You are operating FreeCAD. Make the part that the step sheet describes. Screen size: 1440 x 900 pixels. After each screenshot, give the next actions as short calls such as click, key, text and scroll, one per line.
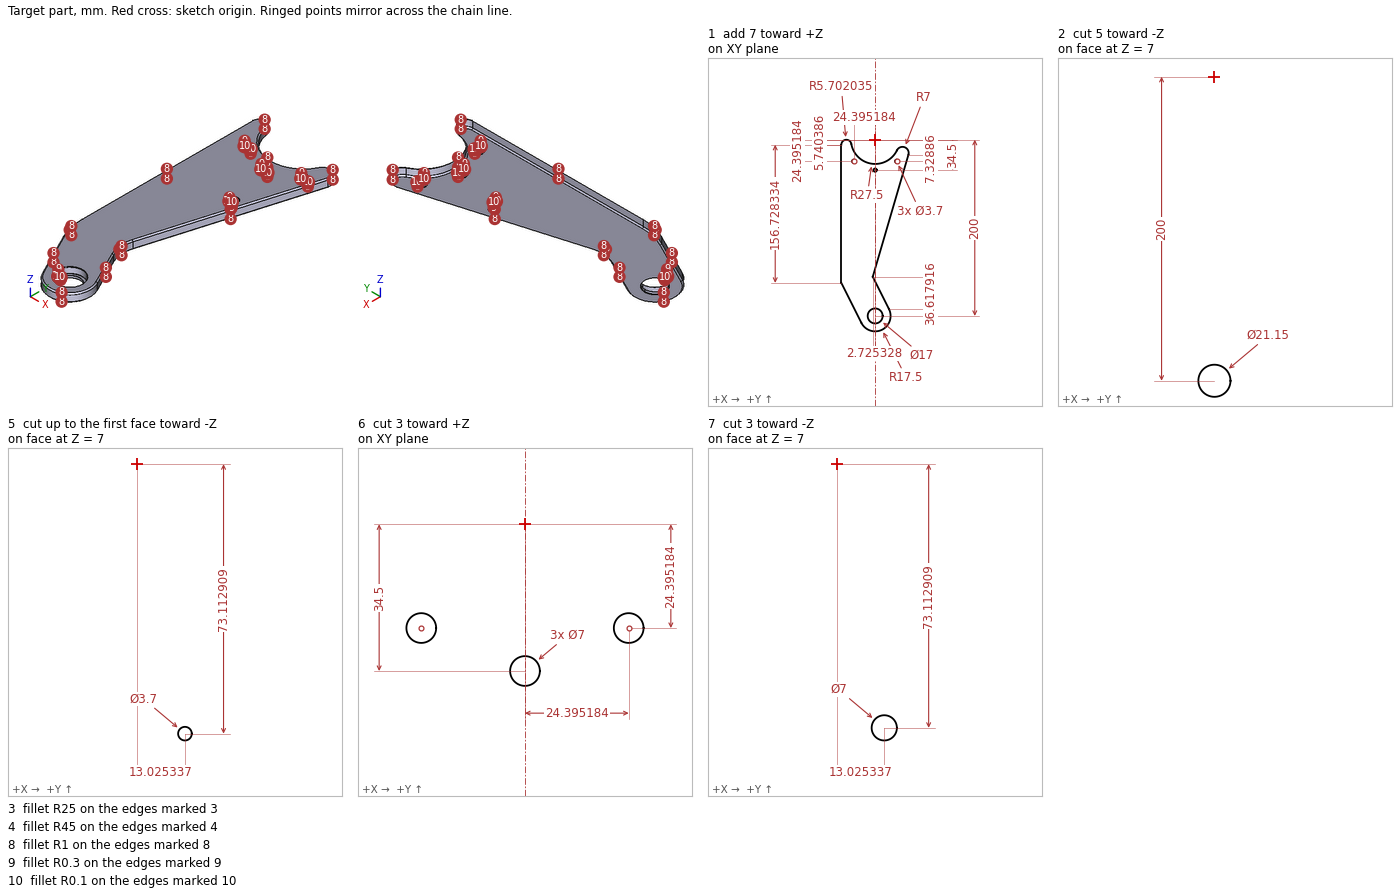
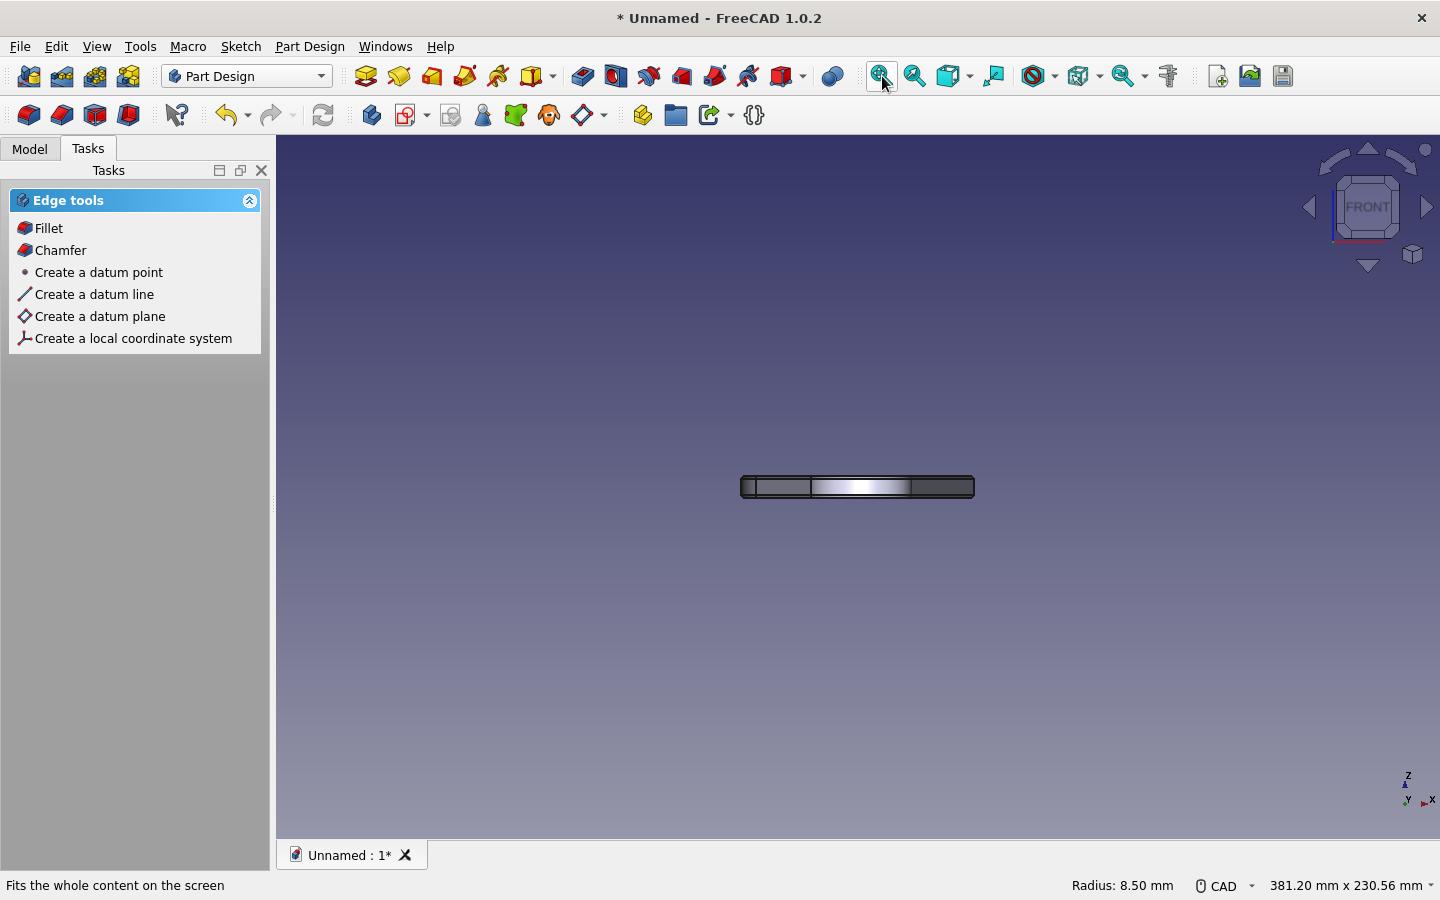
key(3)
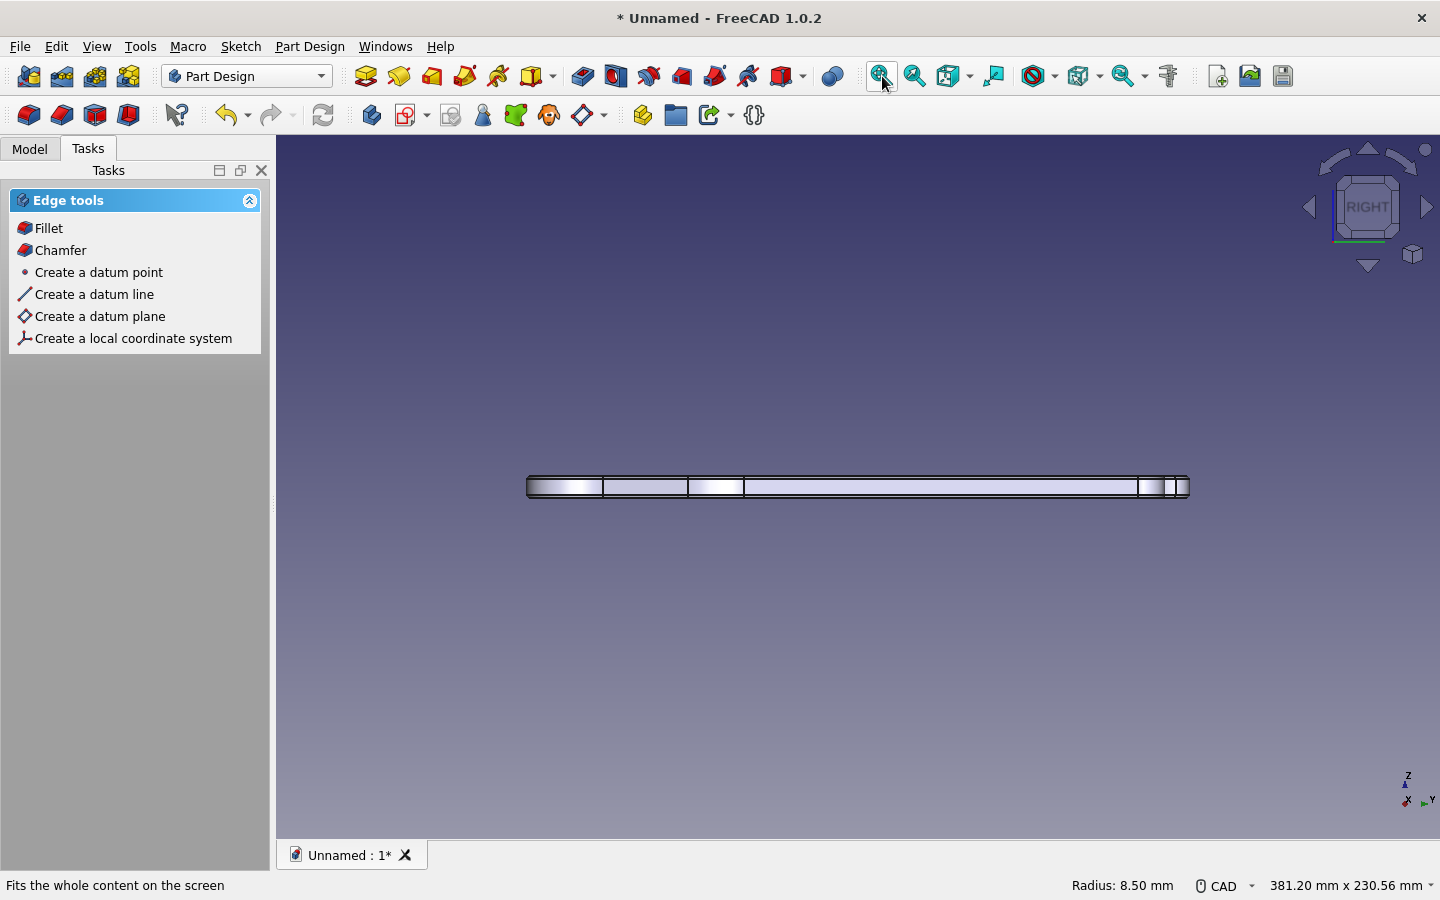
key(5)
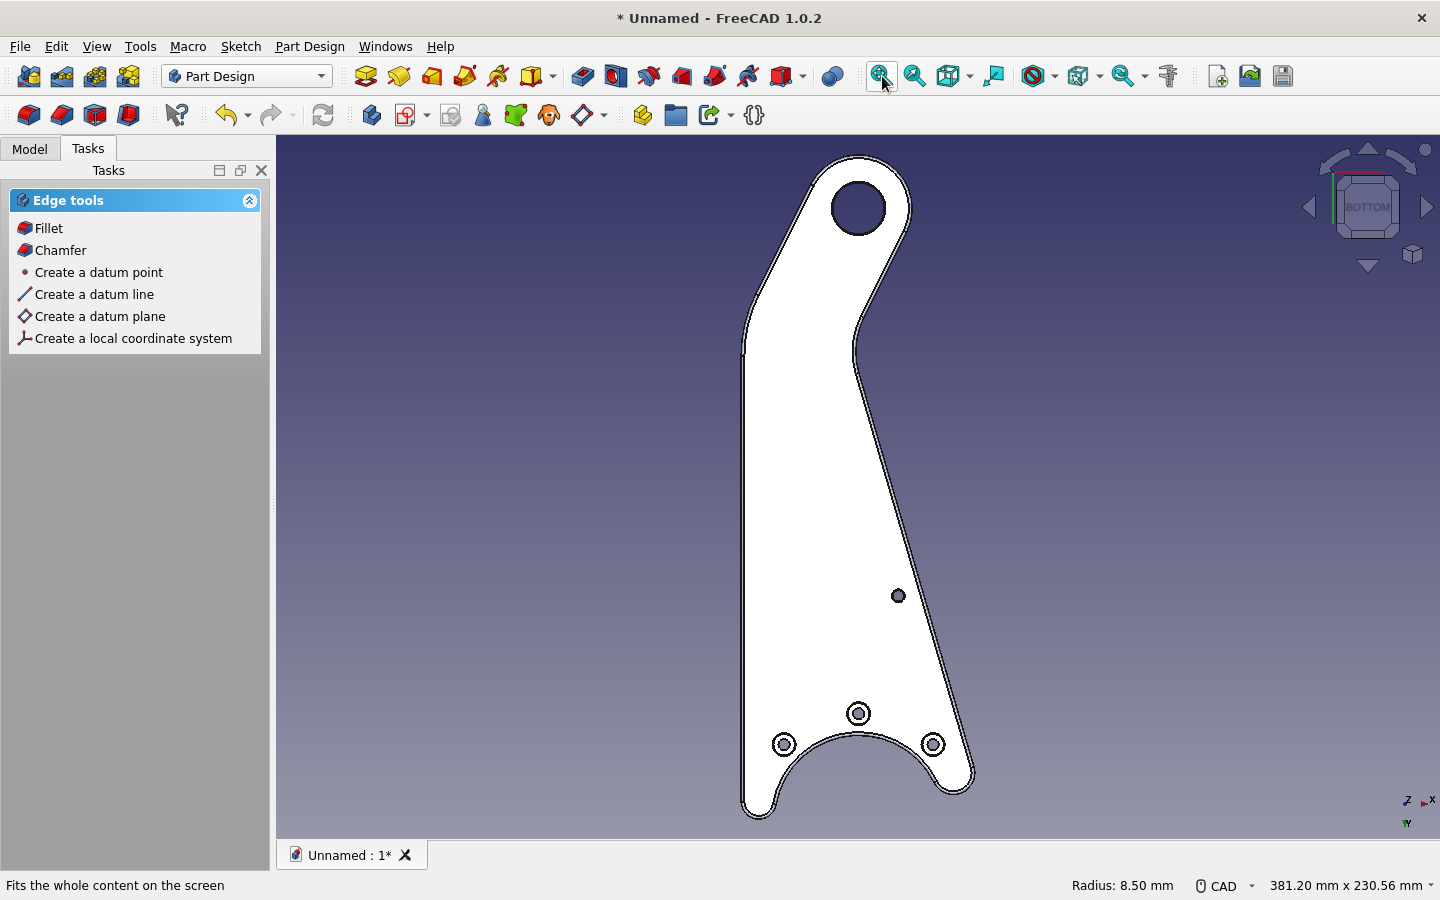
key(4)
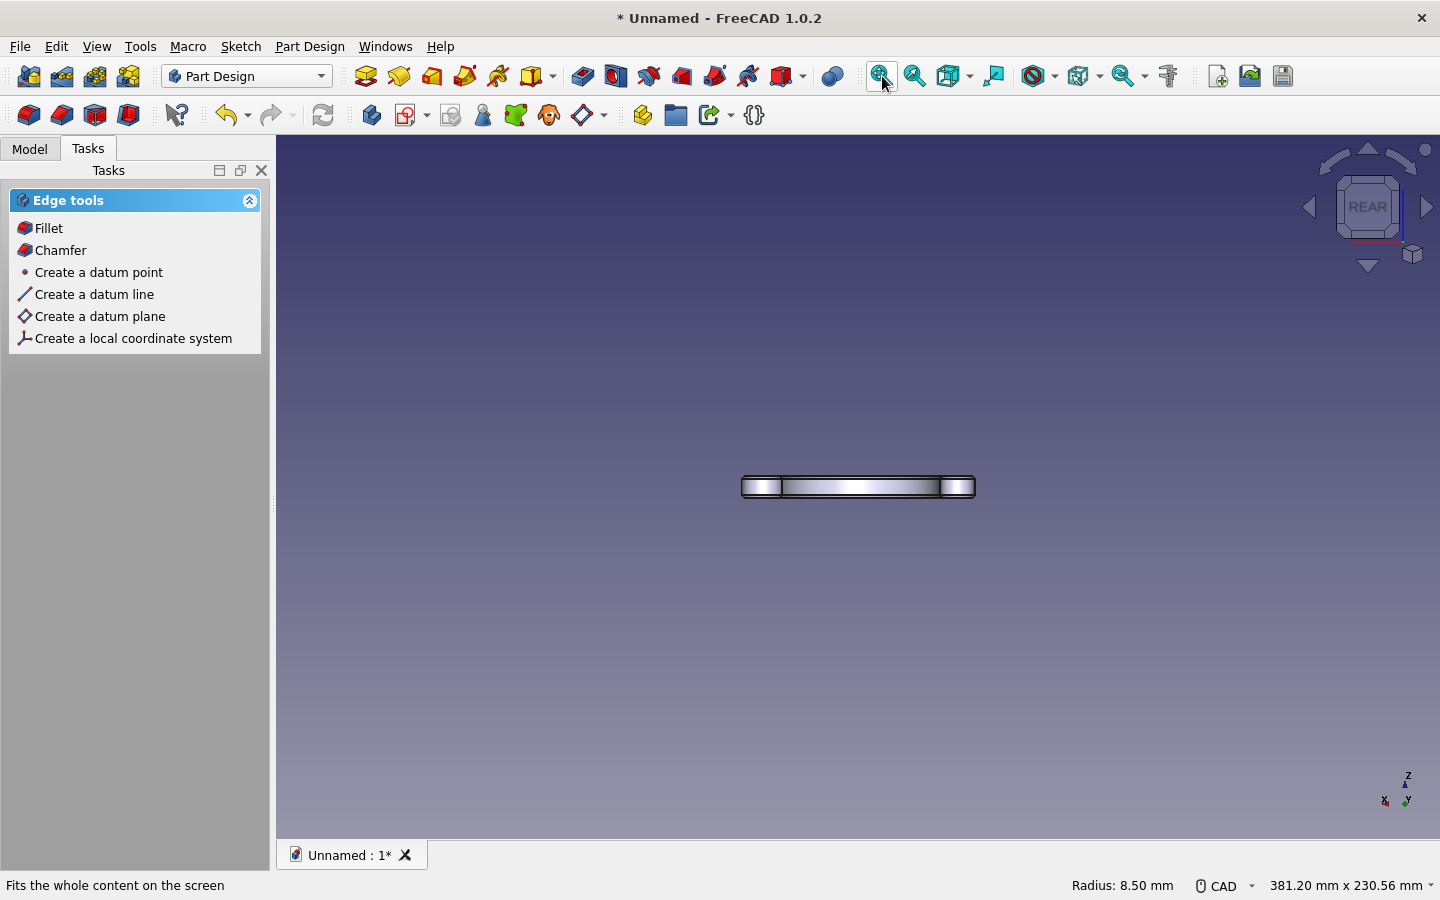
click(882, 76)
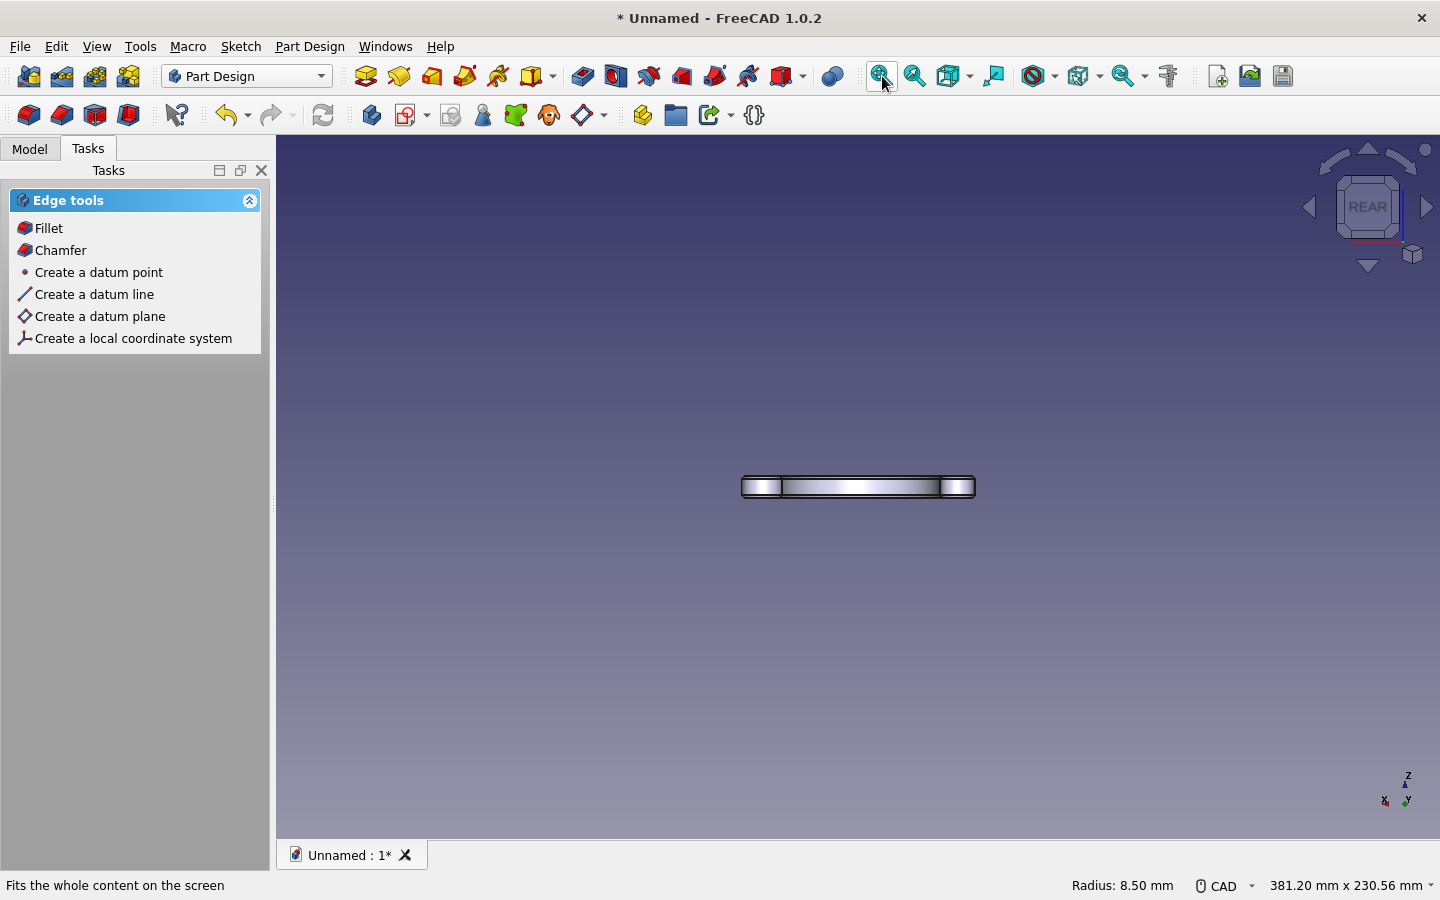
key(6)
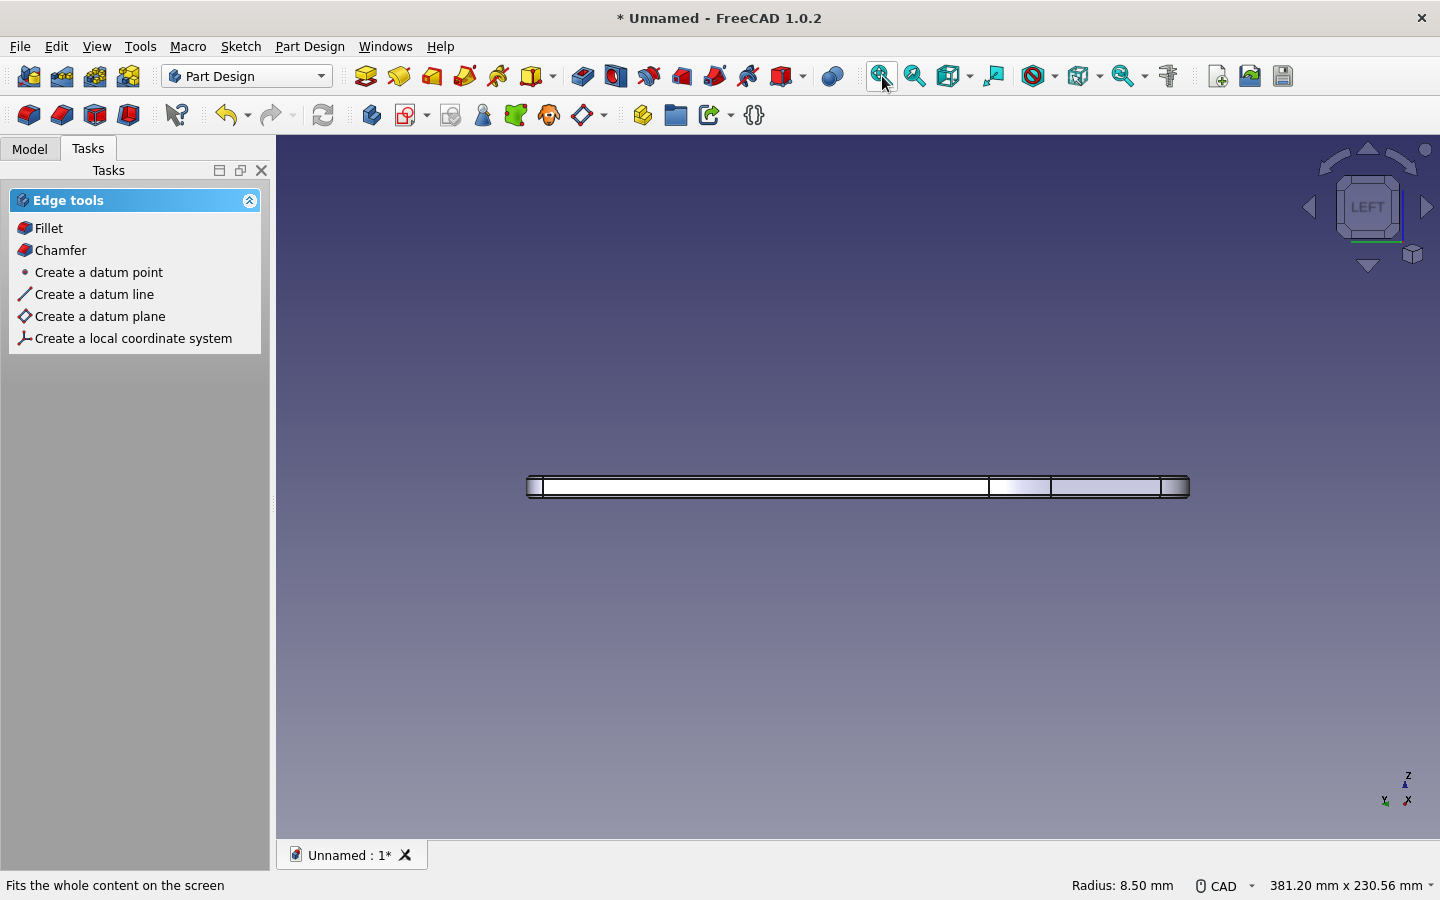
key(v)
key(3)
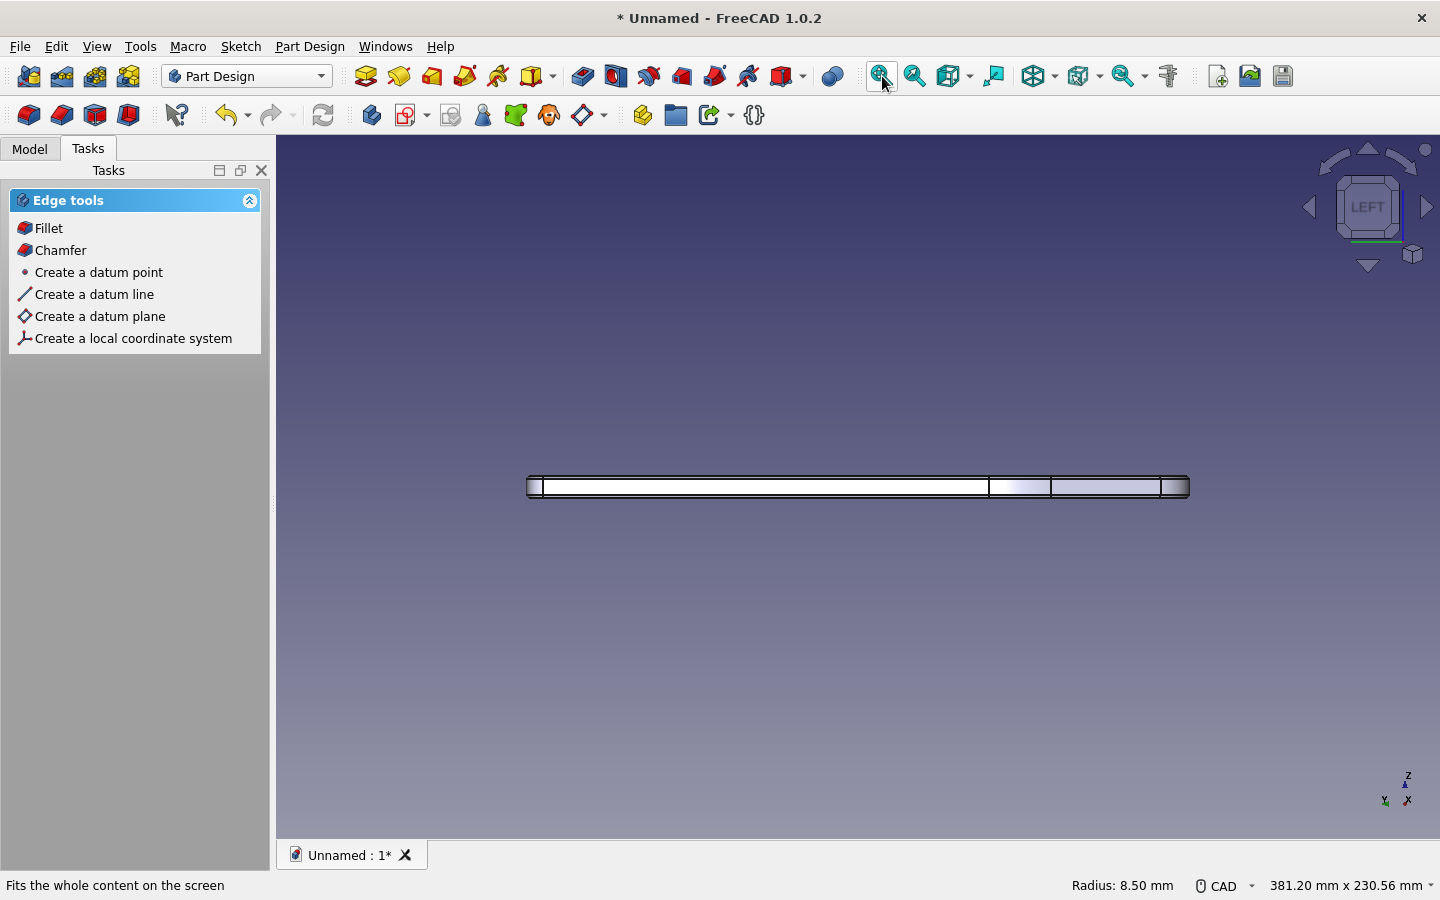
key(0)